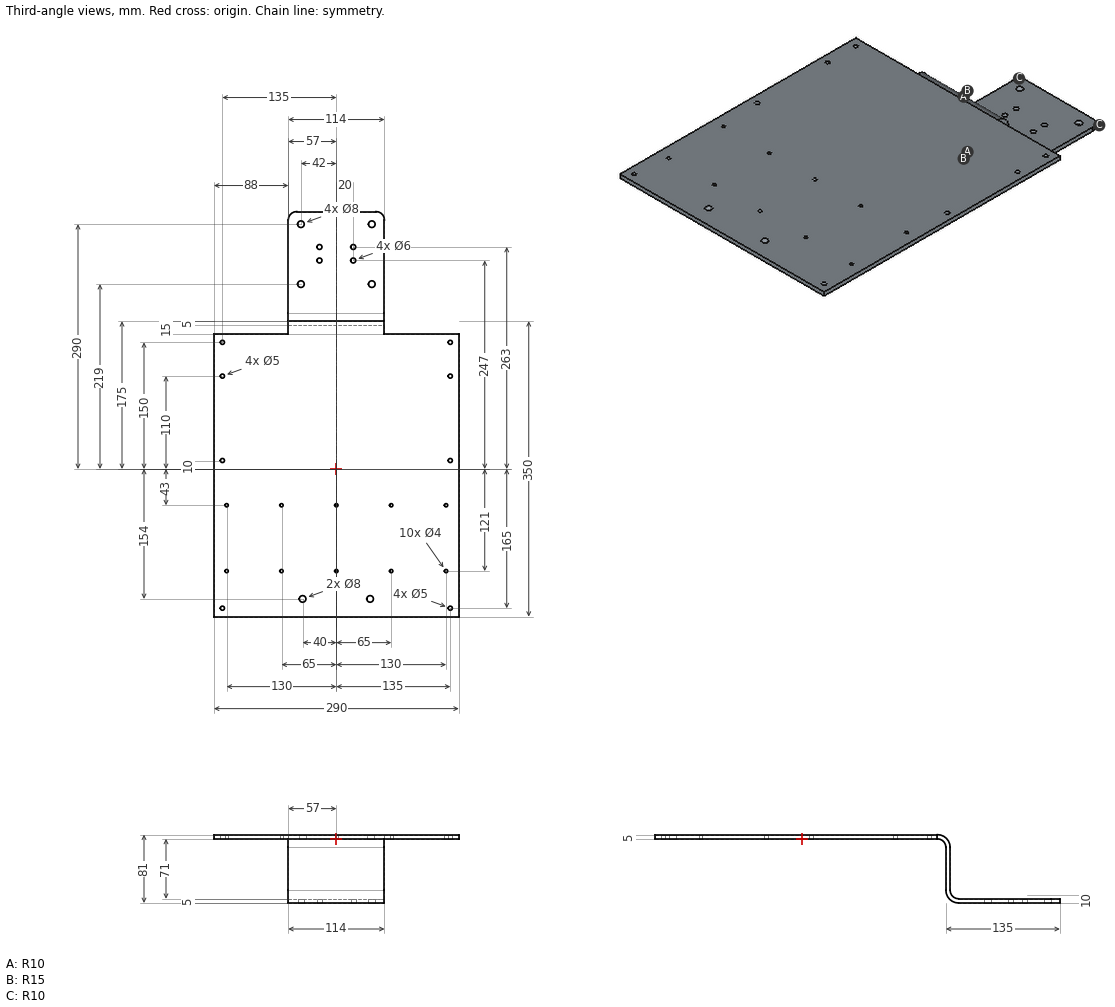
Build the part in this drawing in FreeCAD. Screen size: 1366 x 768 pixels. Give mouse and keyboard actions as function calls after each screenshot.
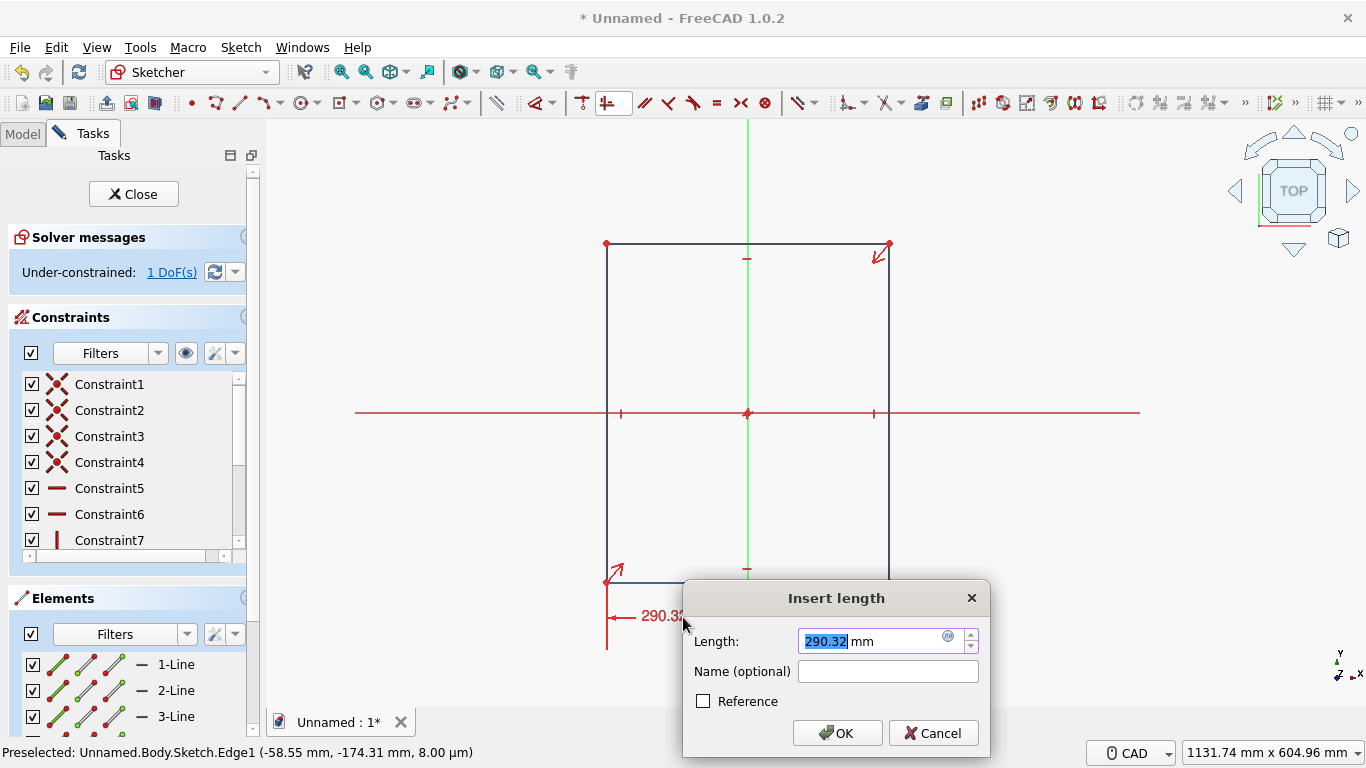
text(290)
key(Return)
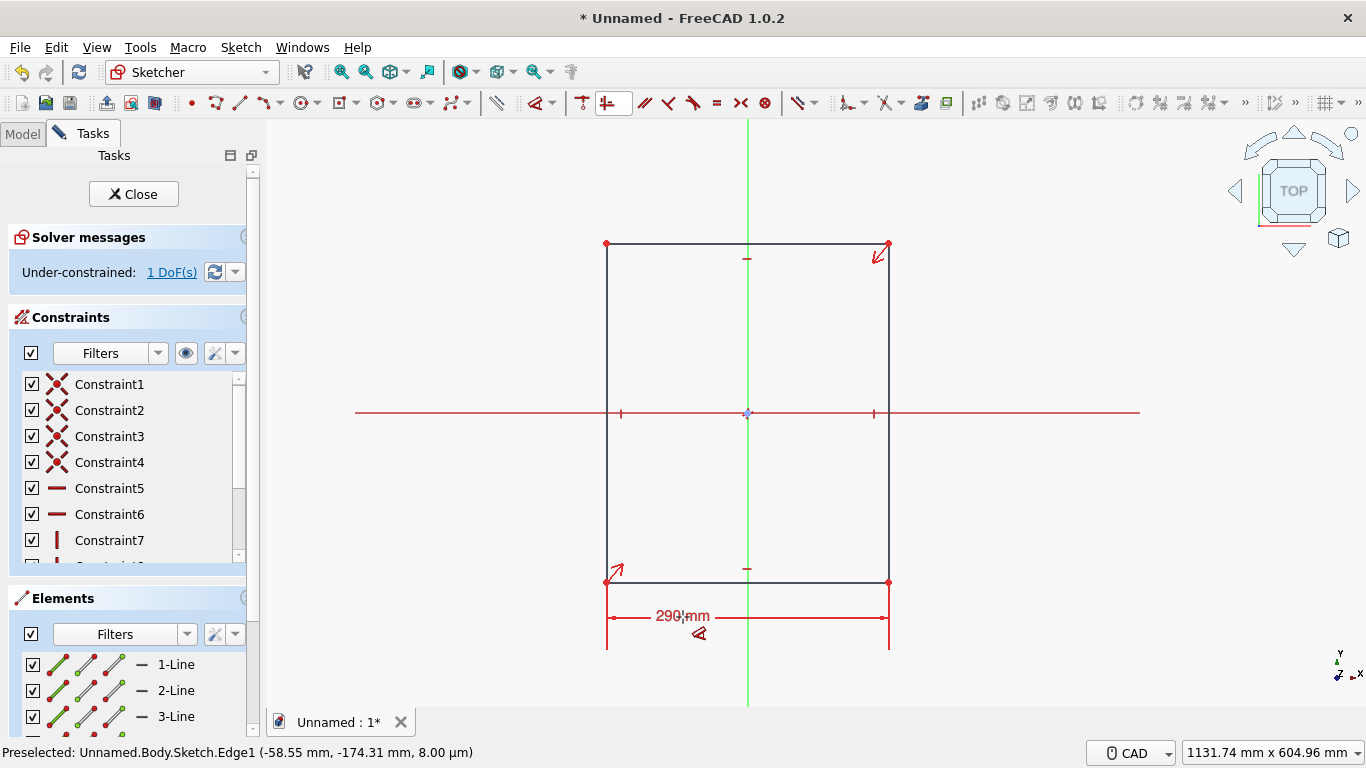
click(889, 481)
click(923, 335)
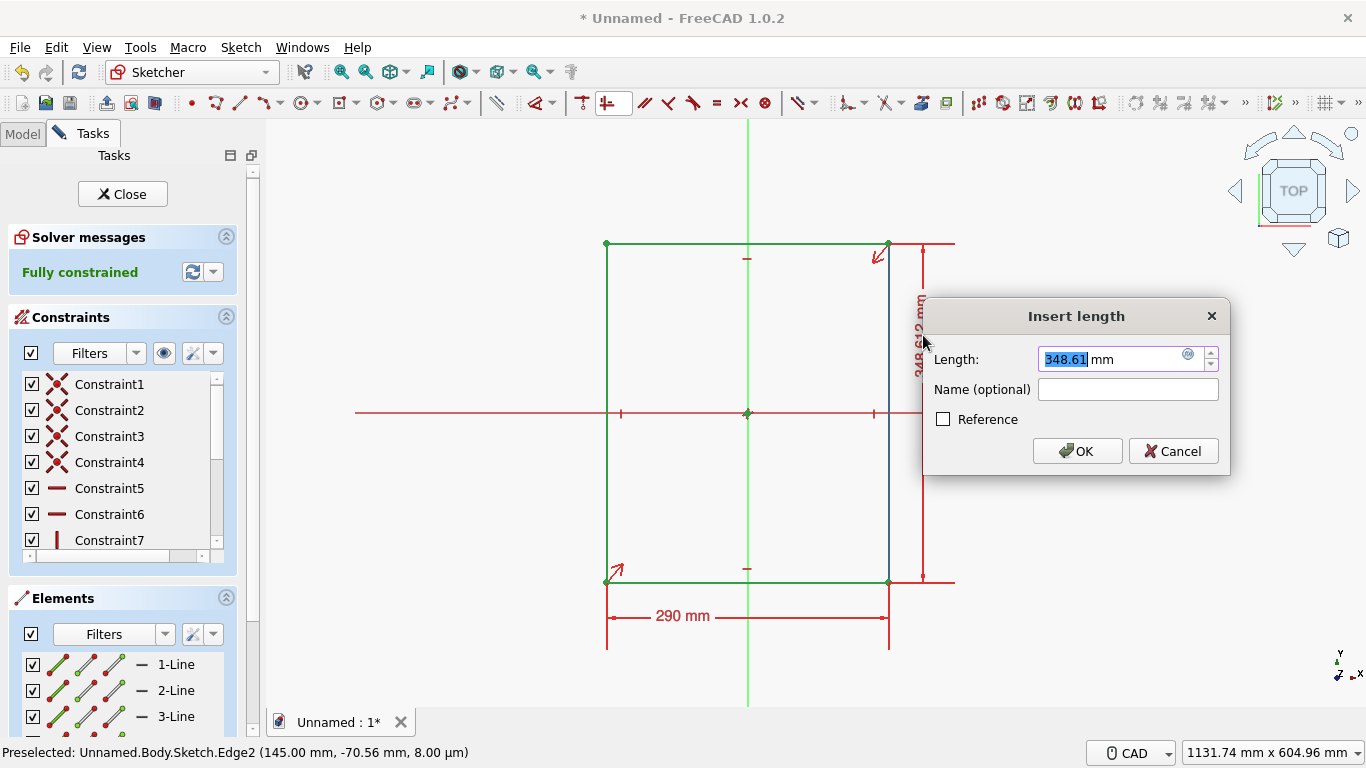
text(350)
key(Return)
key(Escape)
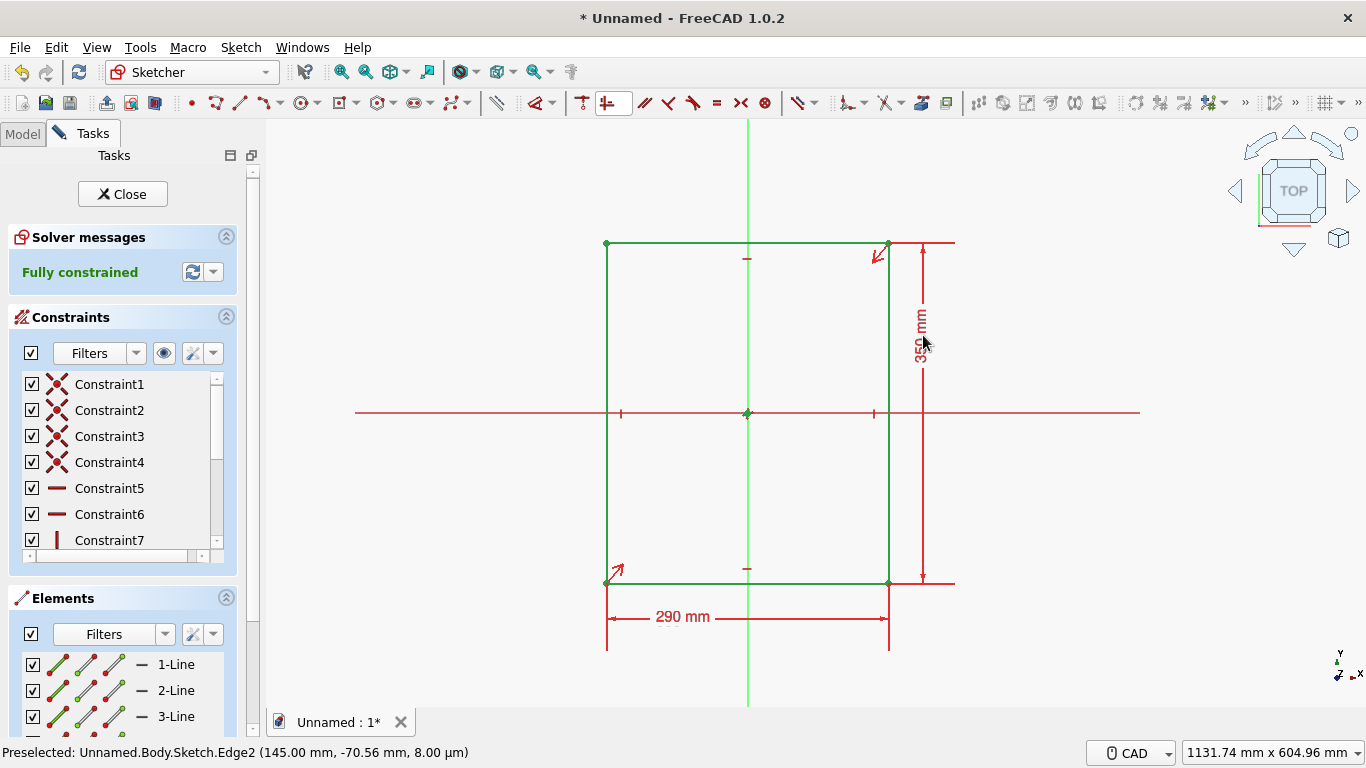
click(123, 194)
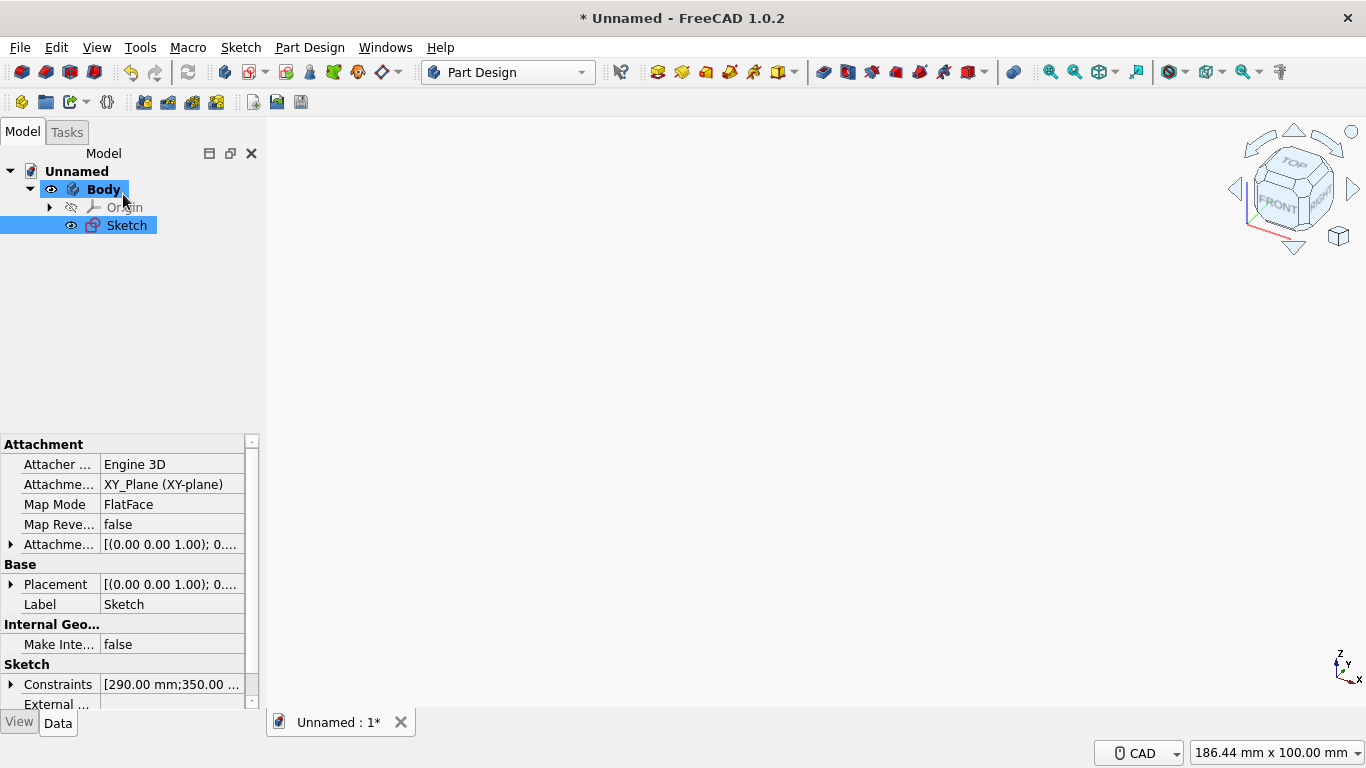
click(658, 72)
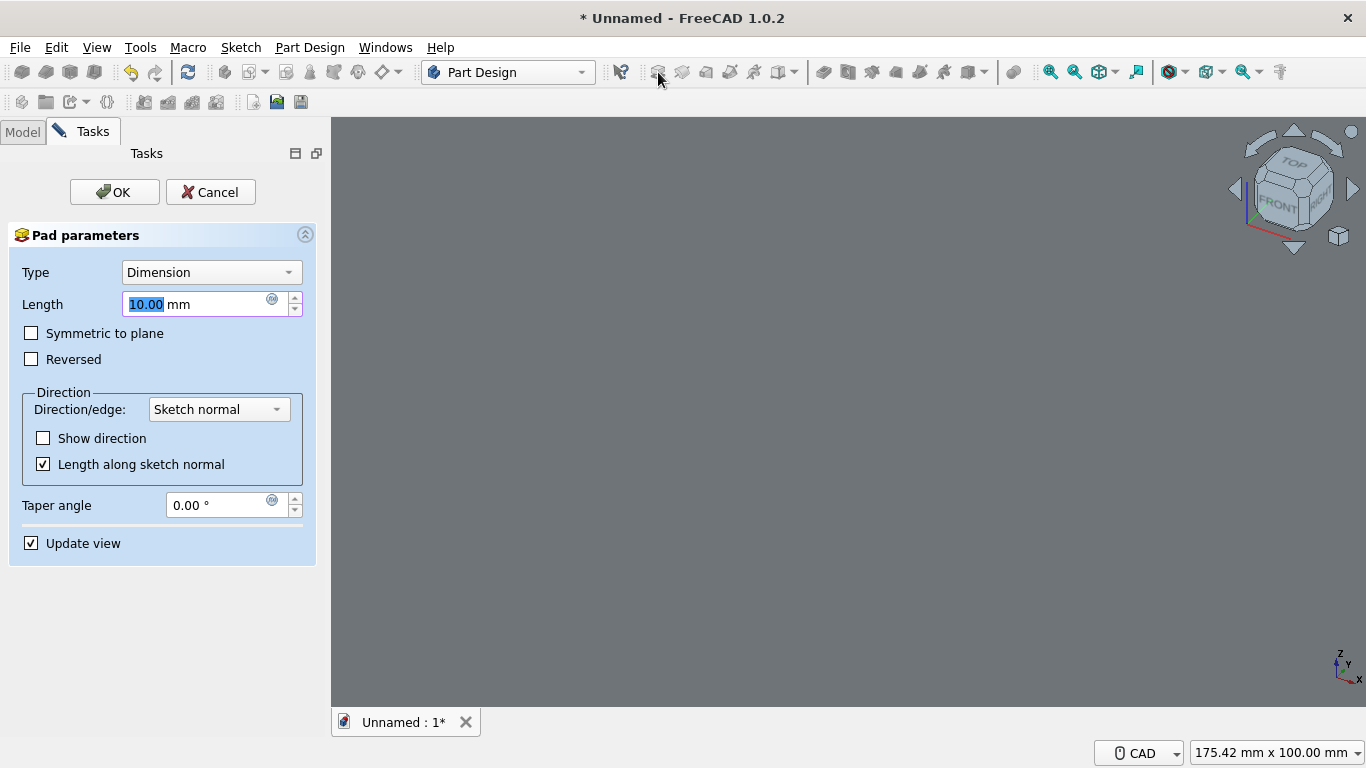
text(5)
key(Tab)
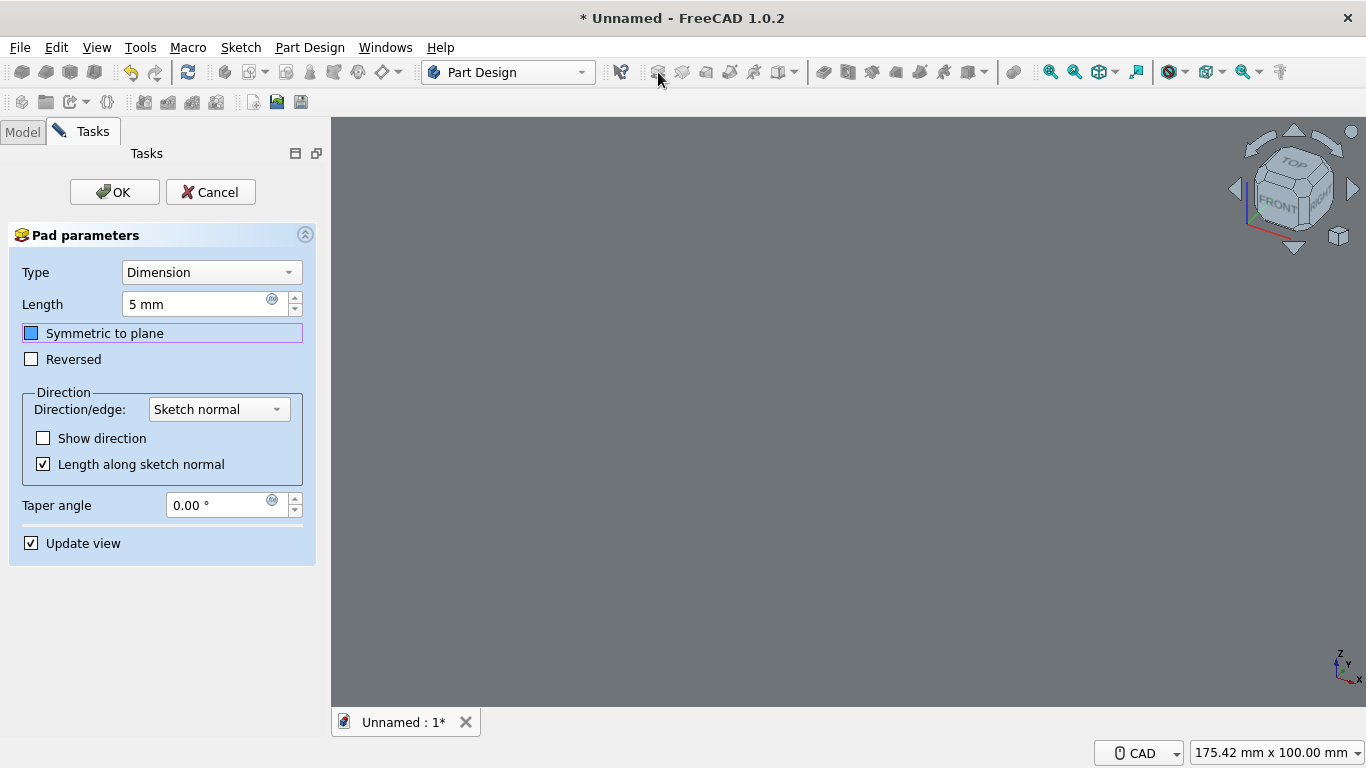
click(115, 192)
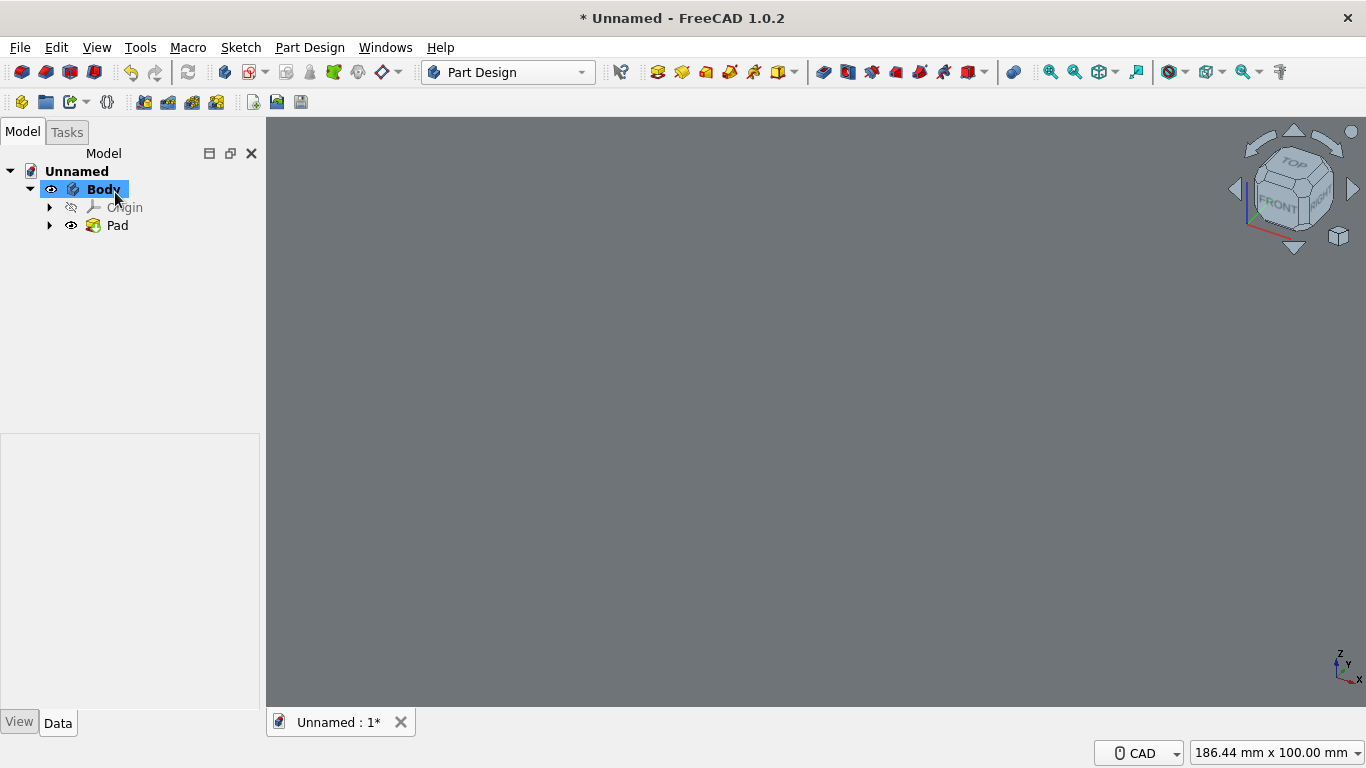
click(1052, 72)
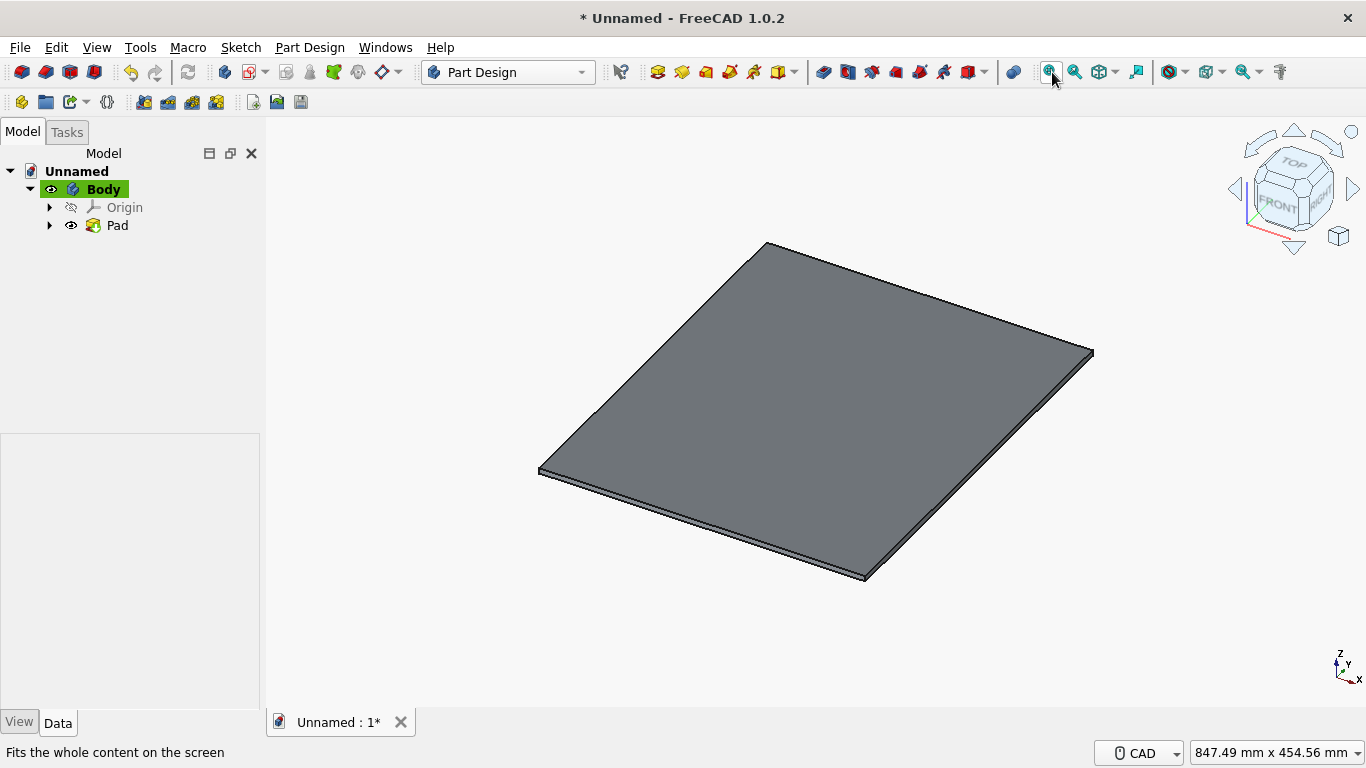
click(816, 408)